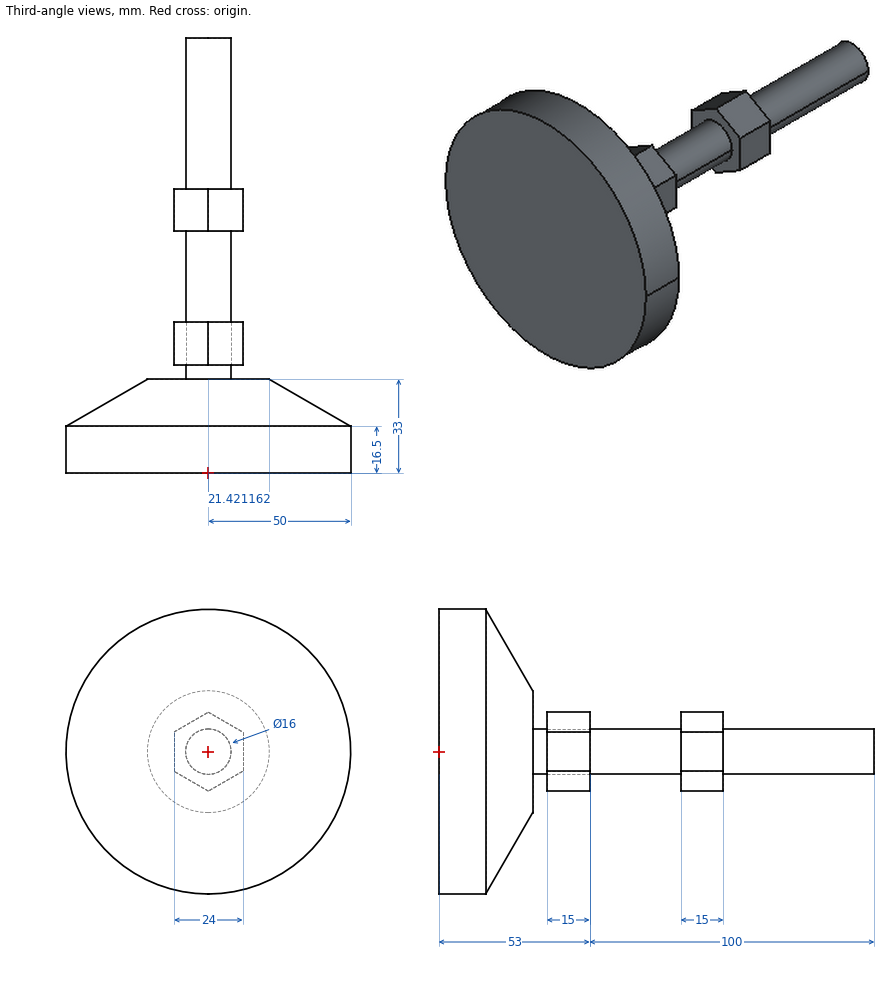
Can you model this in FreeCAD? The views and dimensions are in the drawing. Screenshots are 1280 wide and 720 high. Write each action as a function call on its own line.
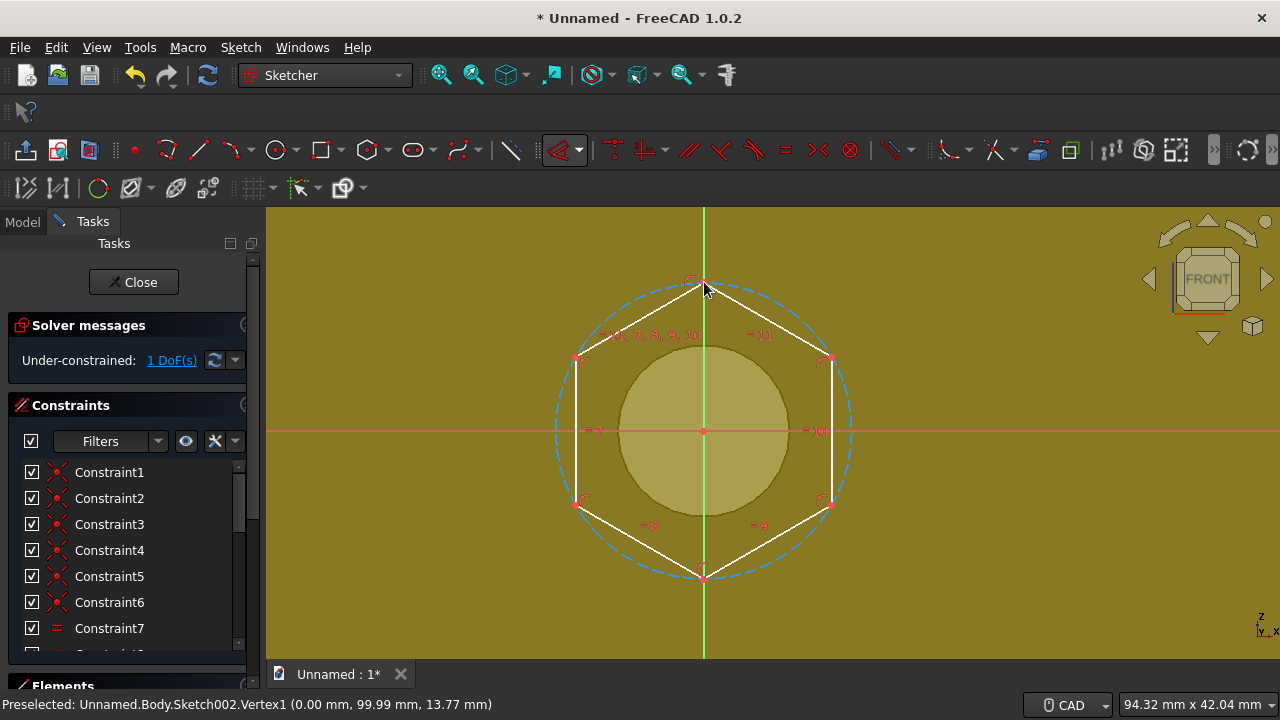
click(576, 357)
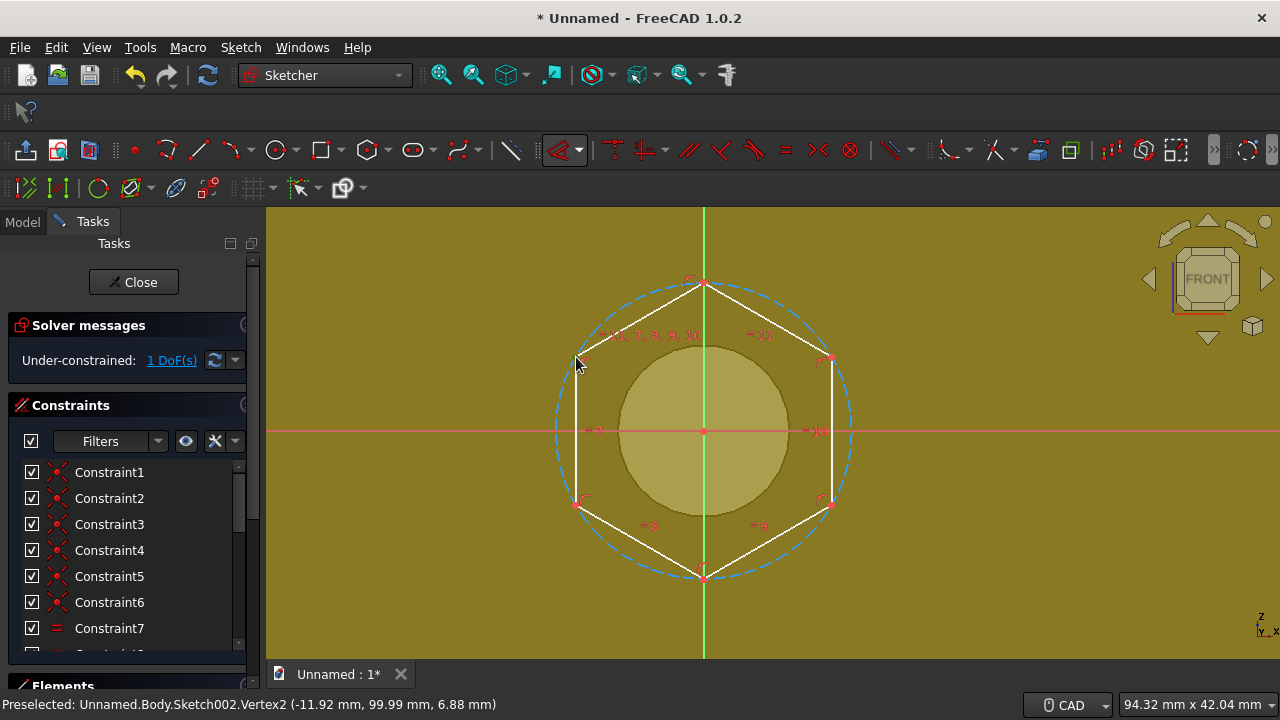
click(832, 505)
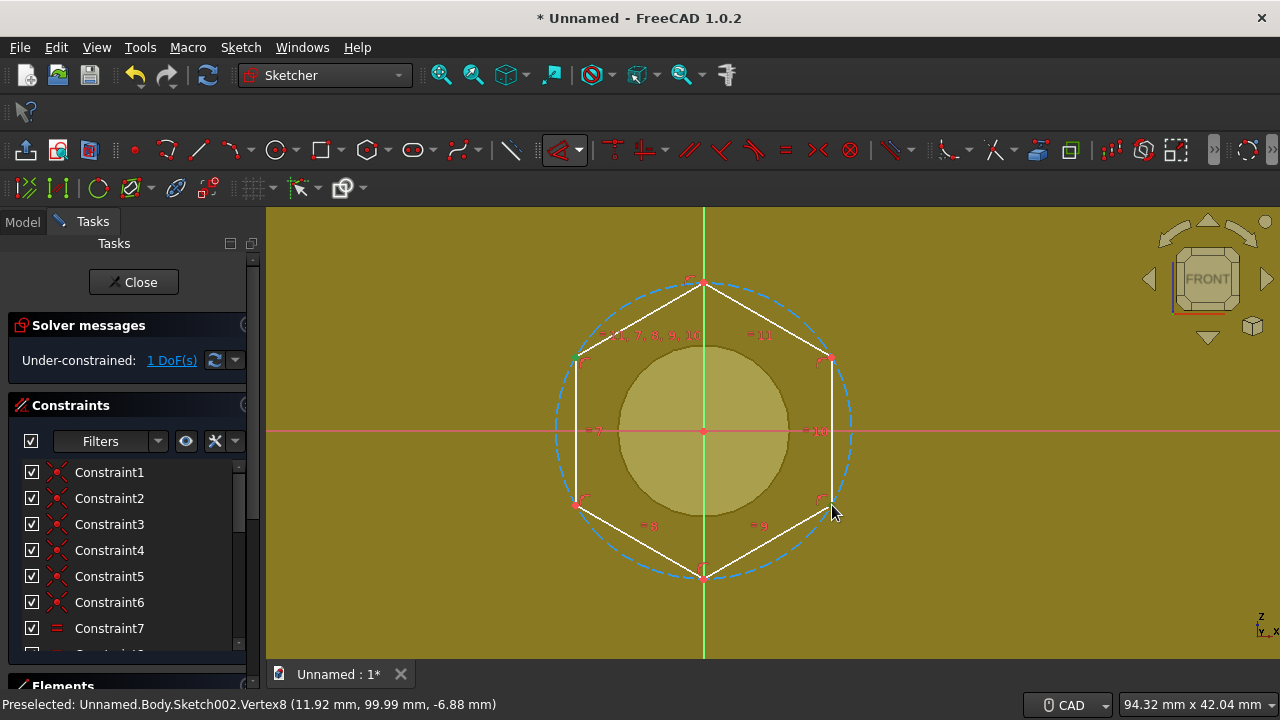
click(582, 150)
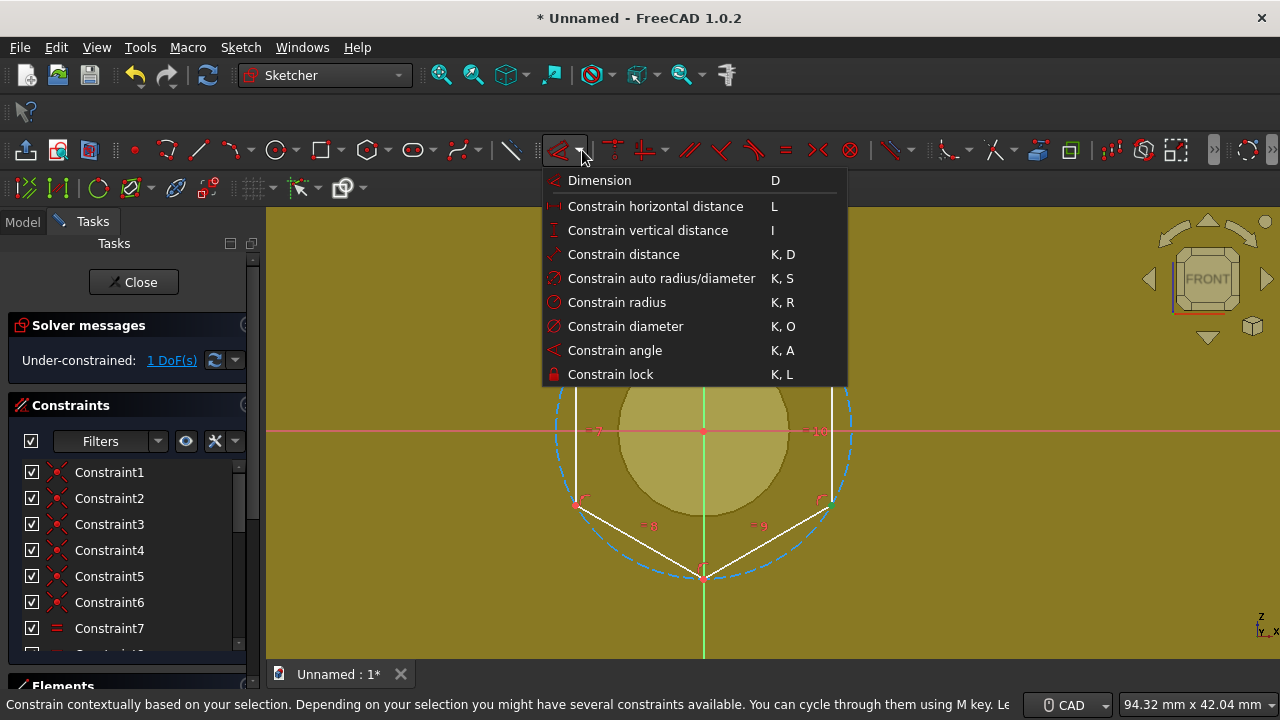
click(695, 206)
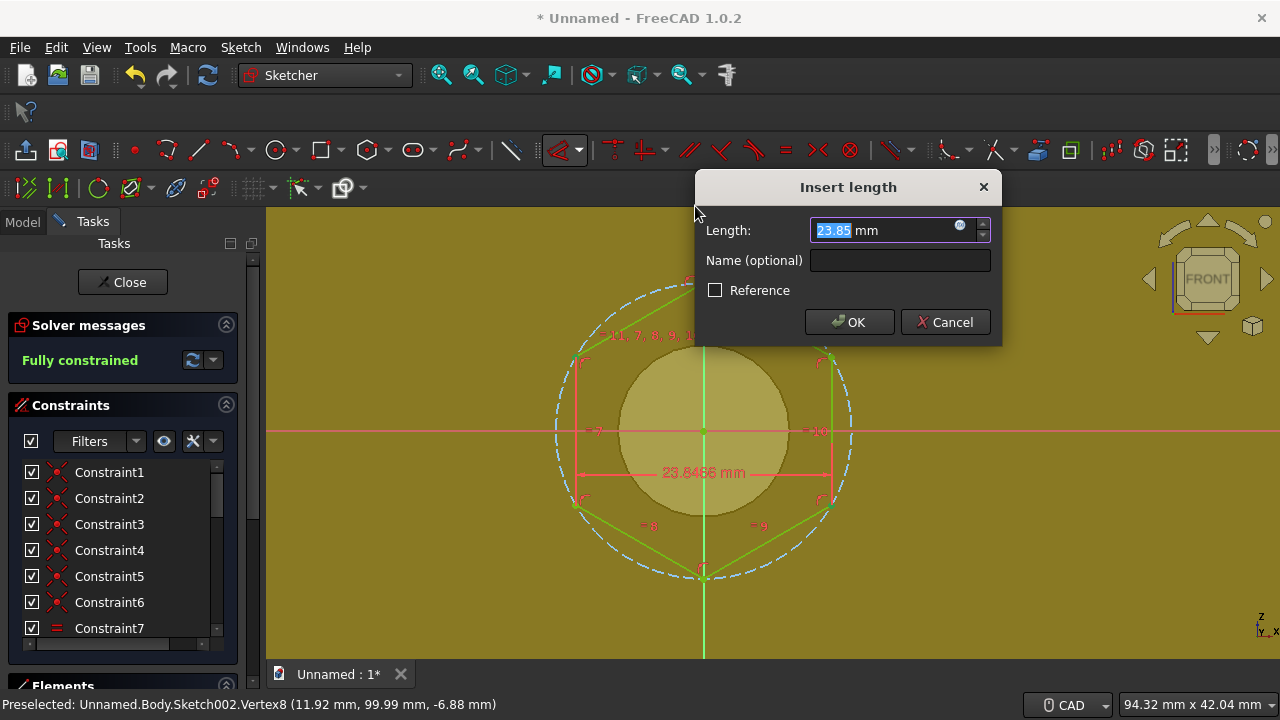
text(24)
key(Return)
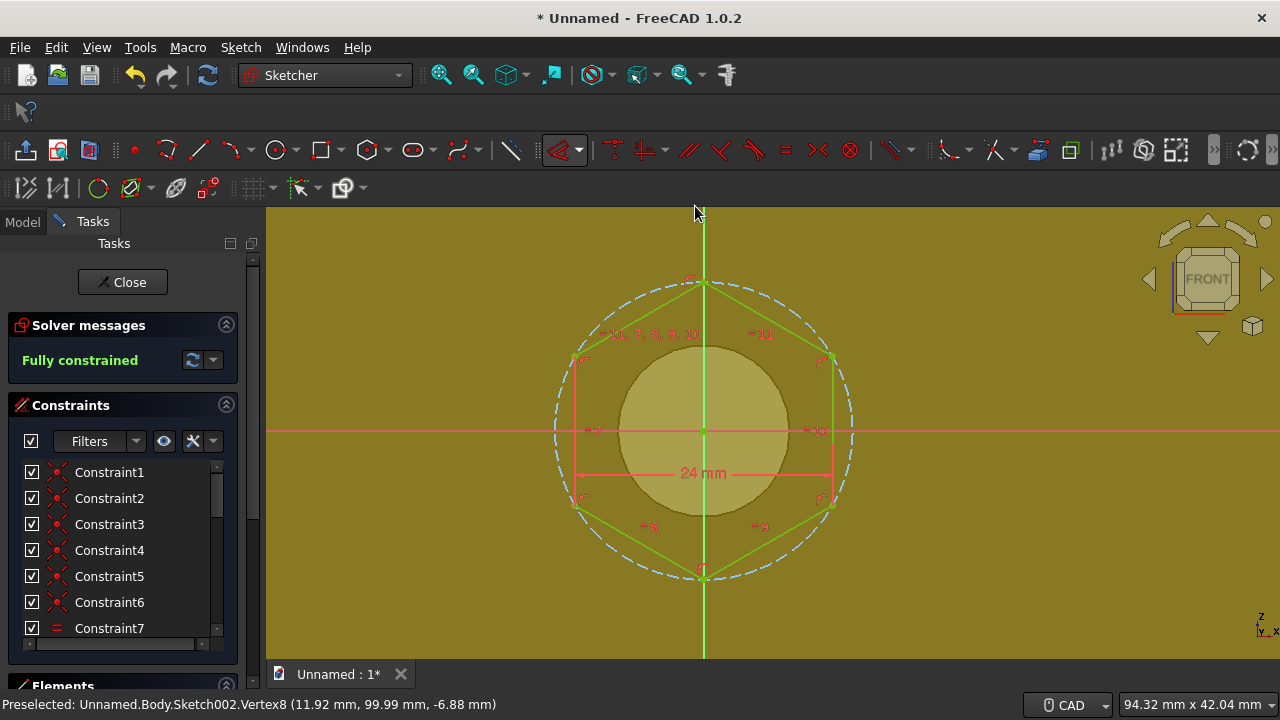
click(123, 282)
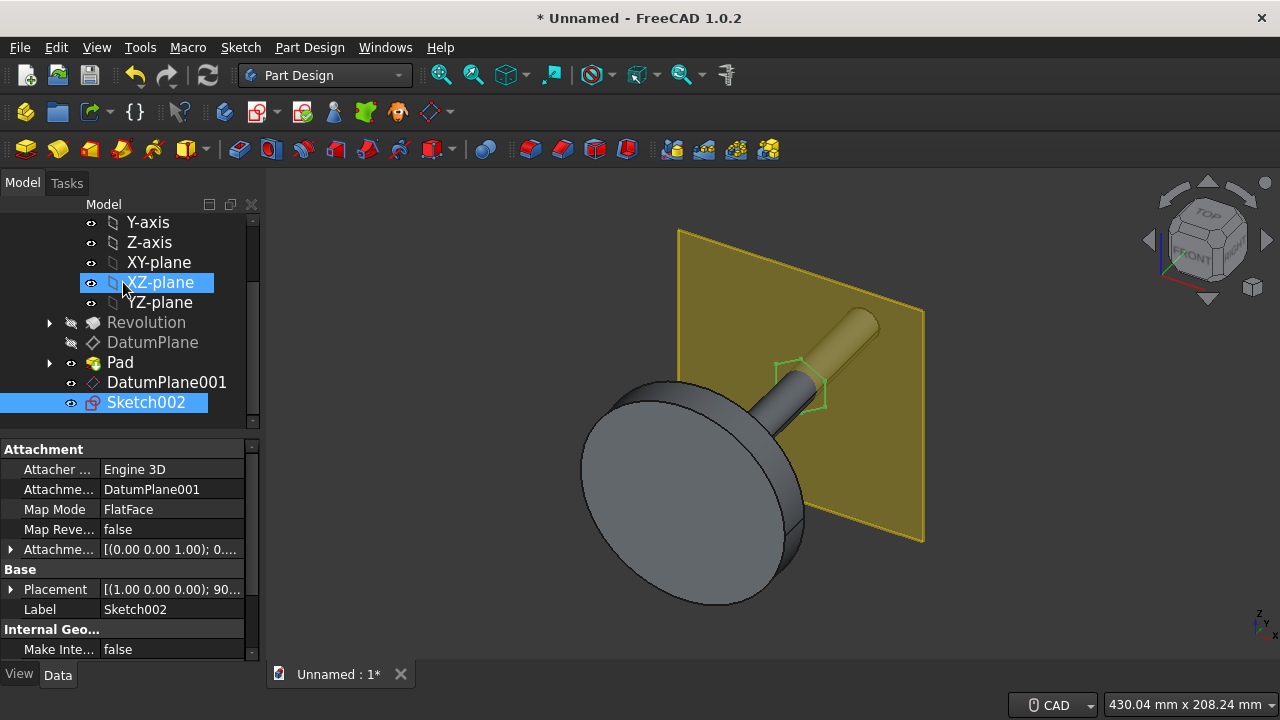
click(26, 150)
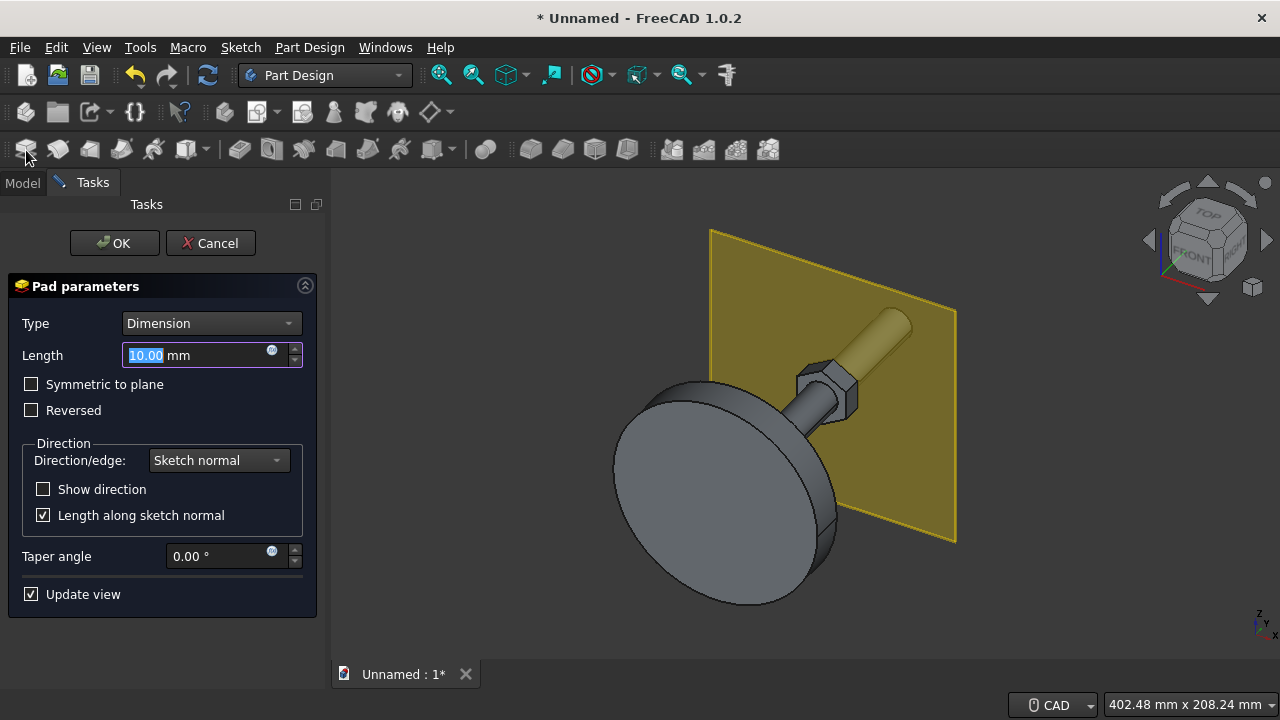
text(15)
key(Tab)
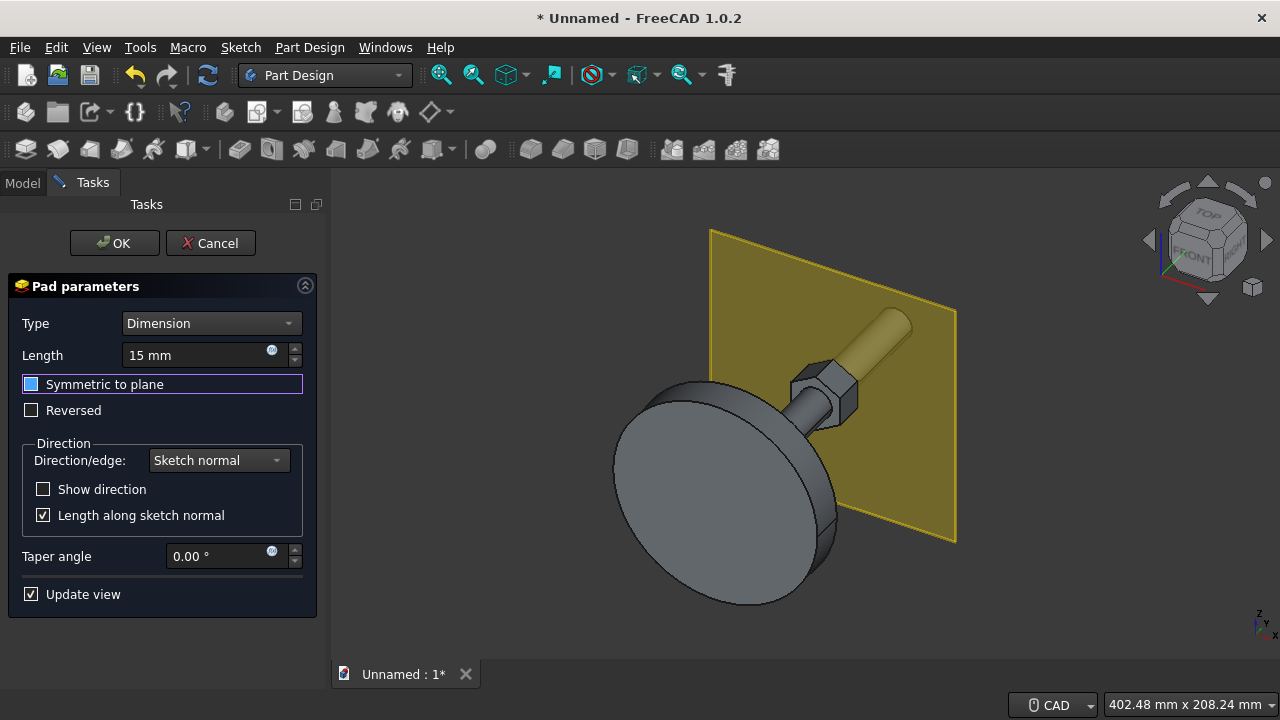
click(115, 243)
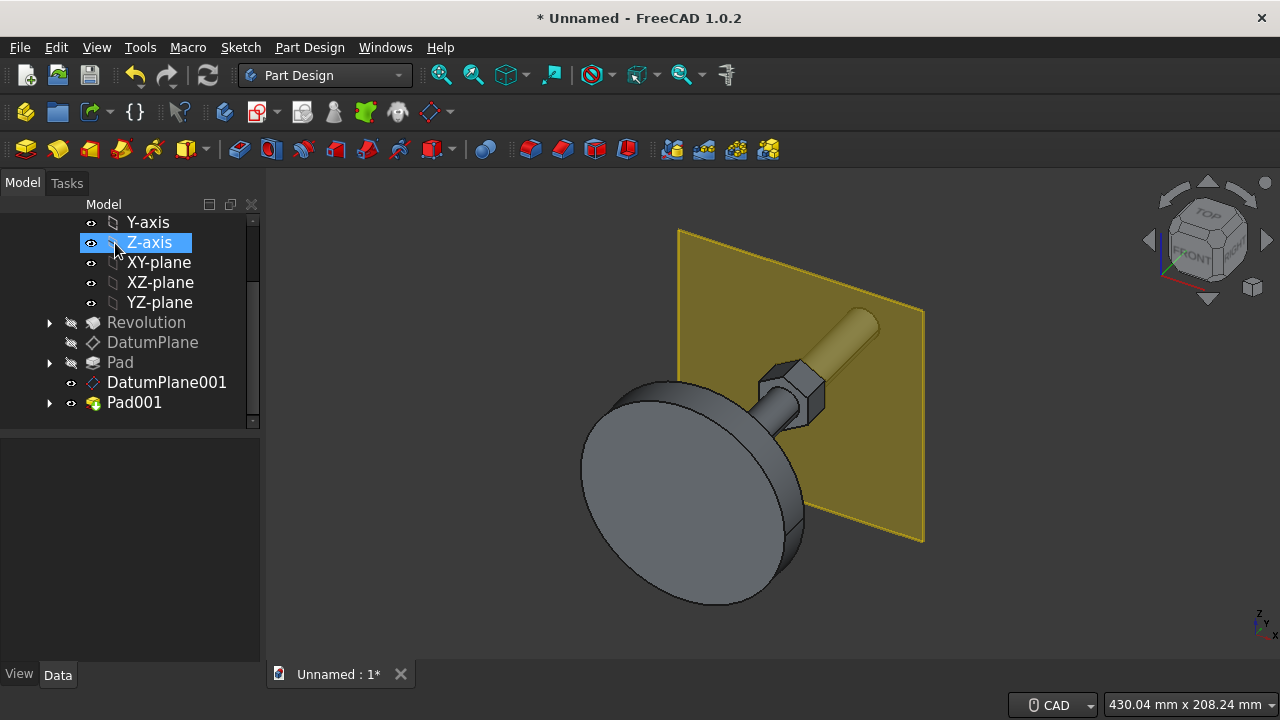
click(116, 383)
key(space)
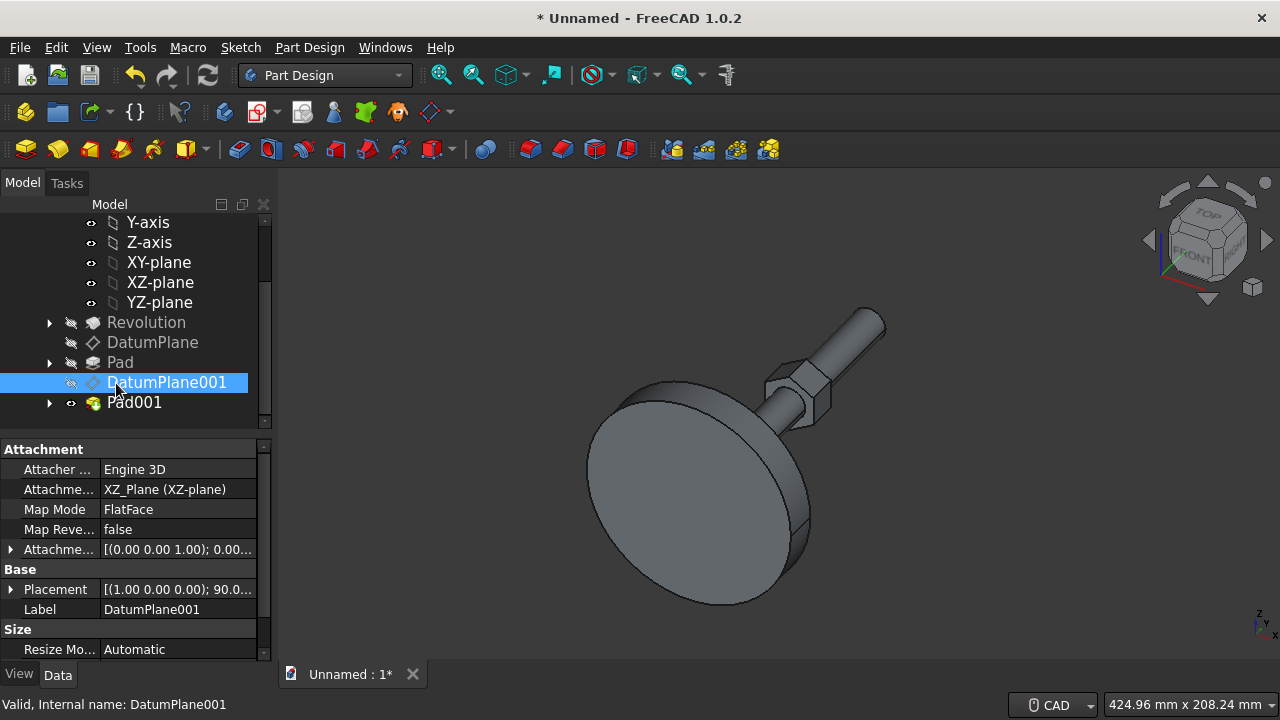
click(318, 619)